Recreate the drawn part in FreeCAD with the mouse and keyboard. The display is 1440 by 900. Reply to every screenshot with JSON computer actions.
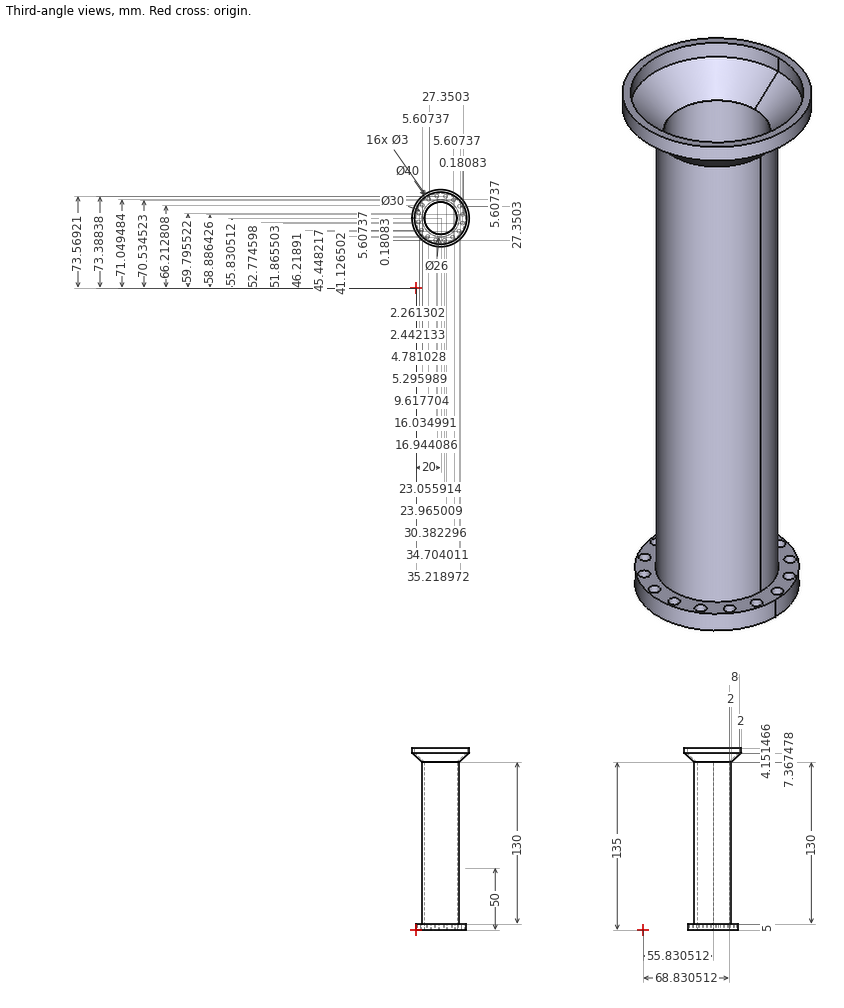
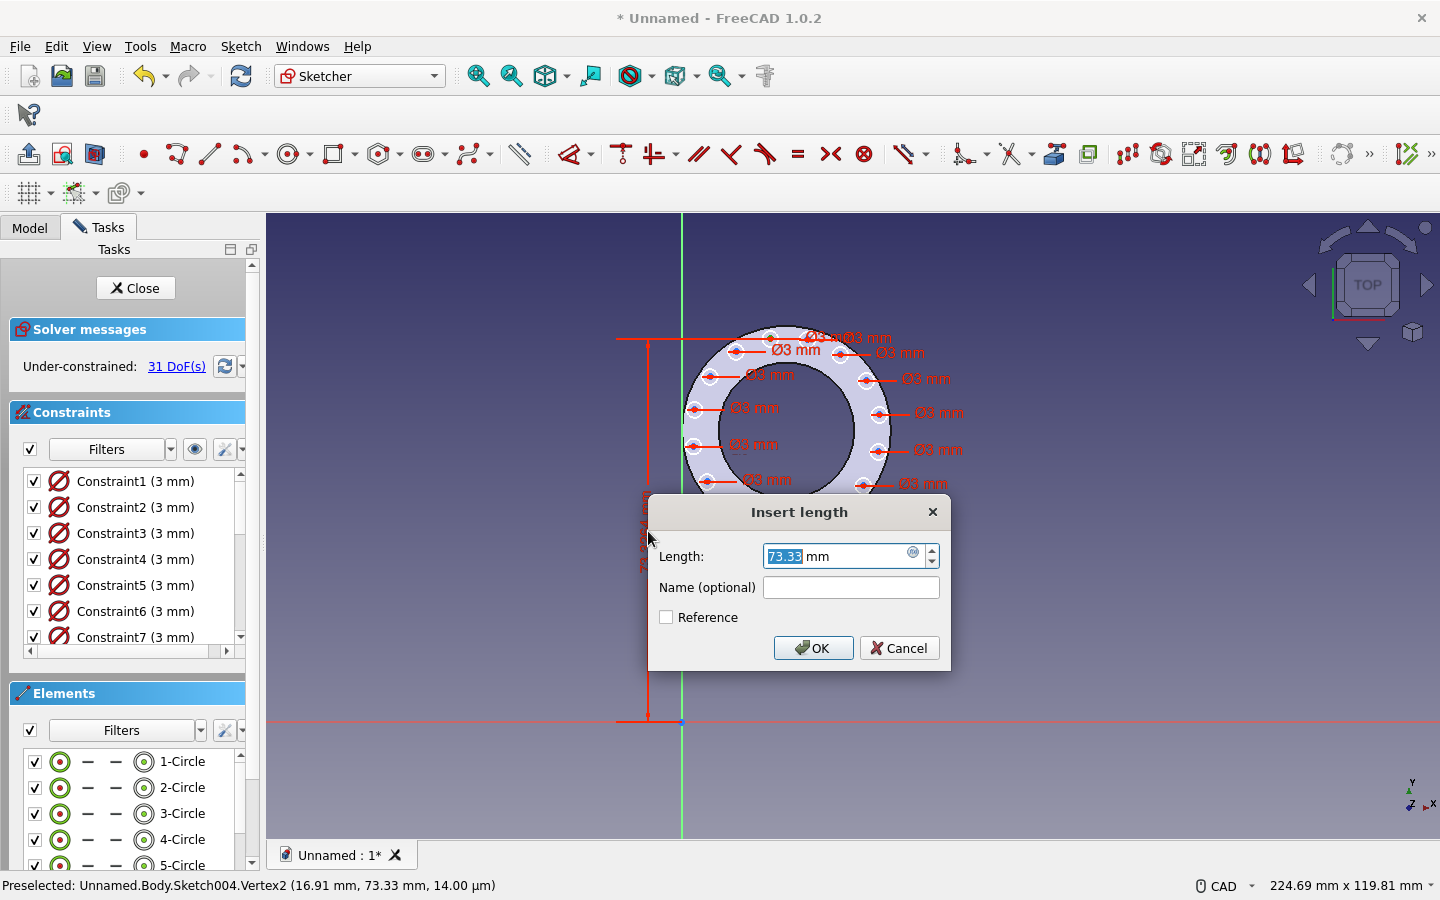
{"action": "type", "text": "73.56921"}
{"action": "key", "text": "Return"}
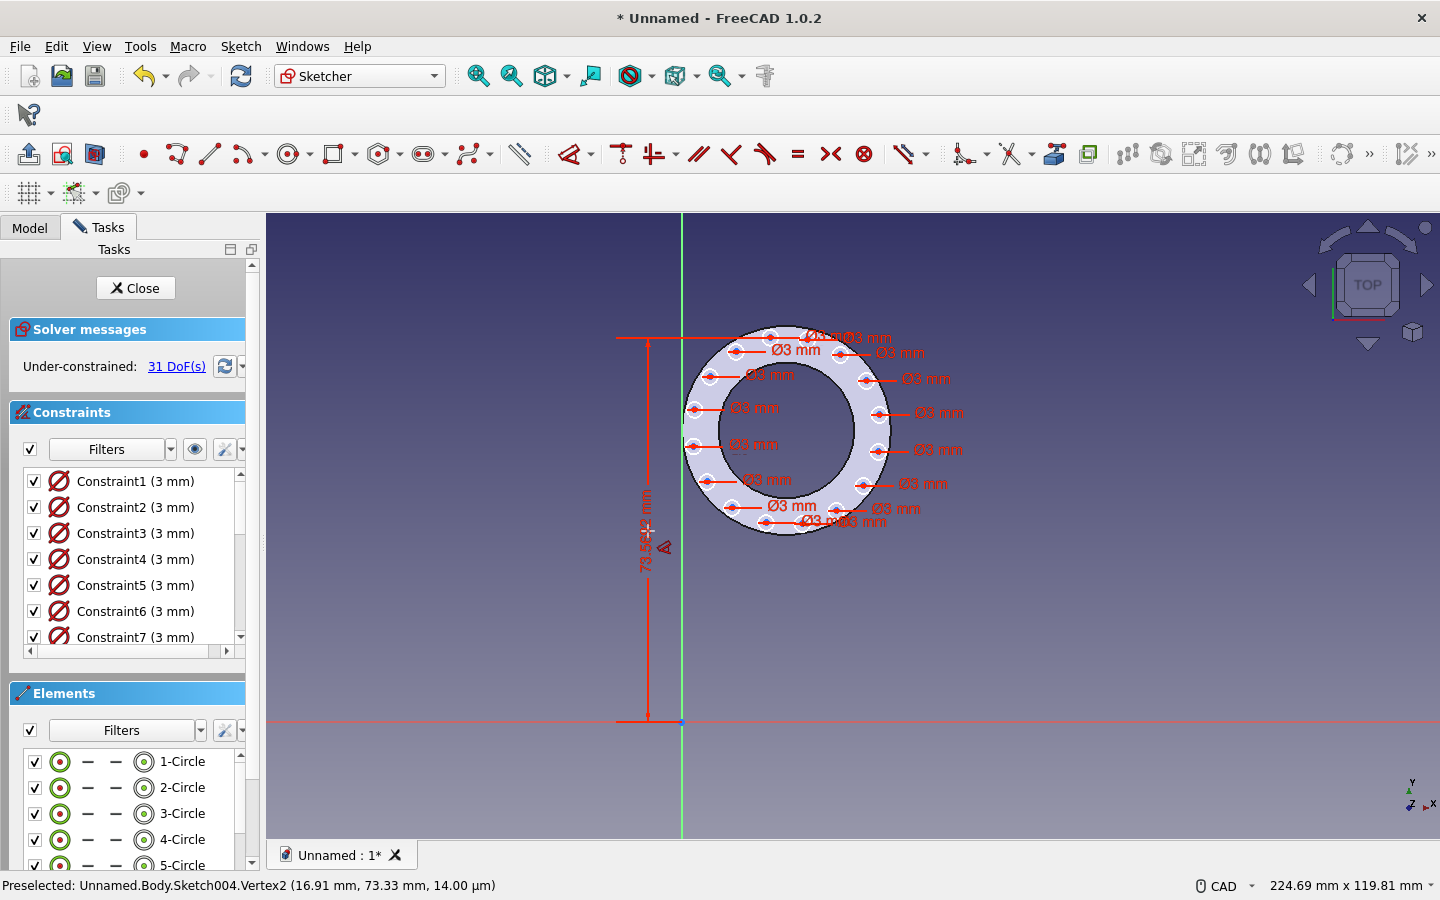
{"action": "left_click", "coordinate": [807, 340]}
{"action": "left_click", "coordinate": [648, 443]}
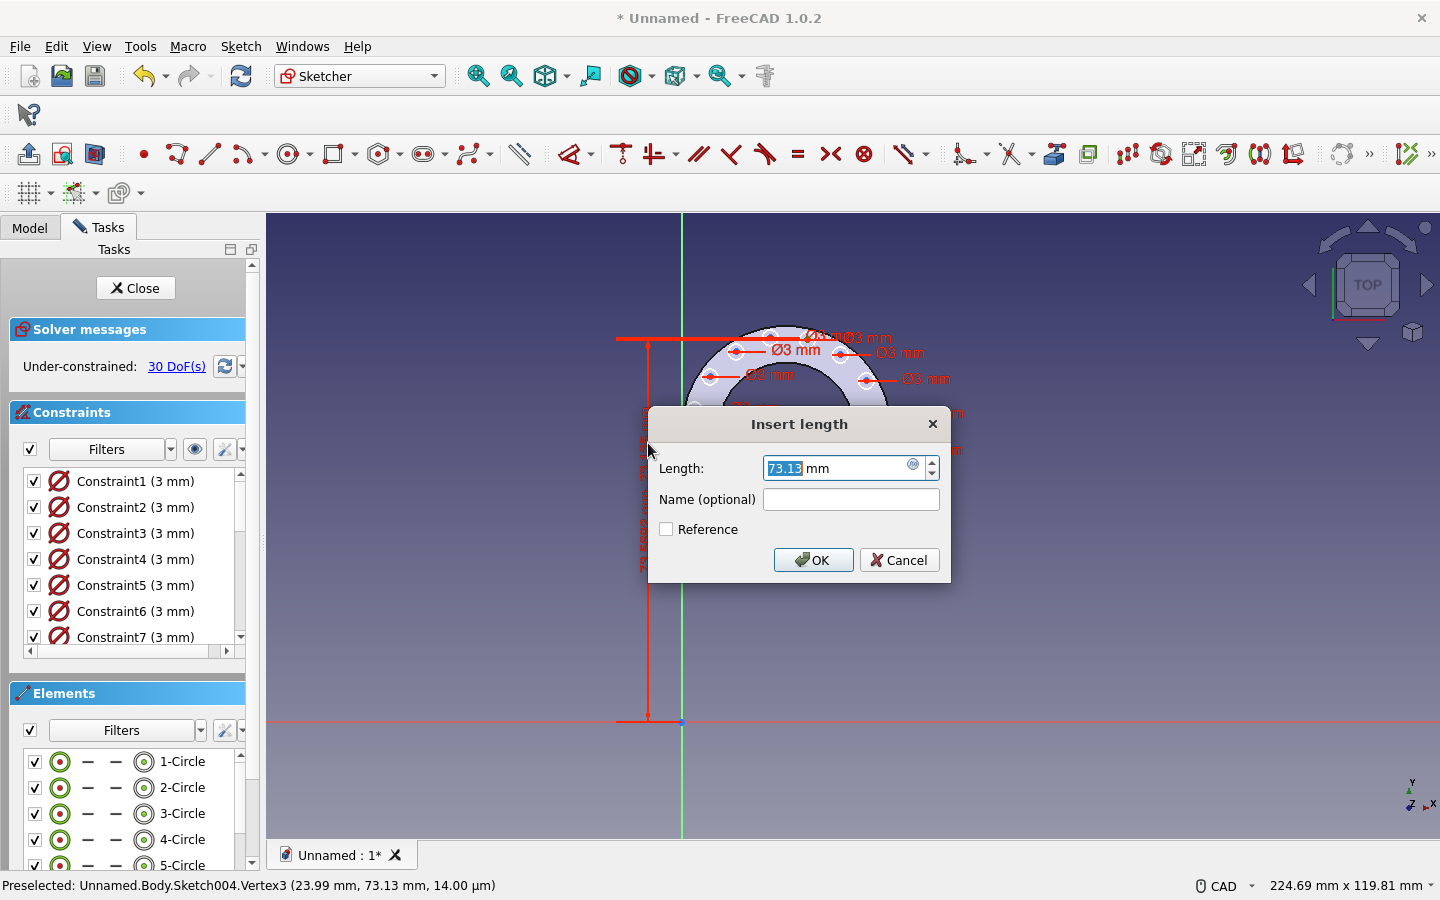
{"action": "type", "text": "73.38838"}
{"action": "key", "text": "Return"}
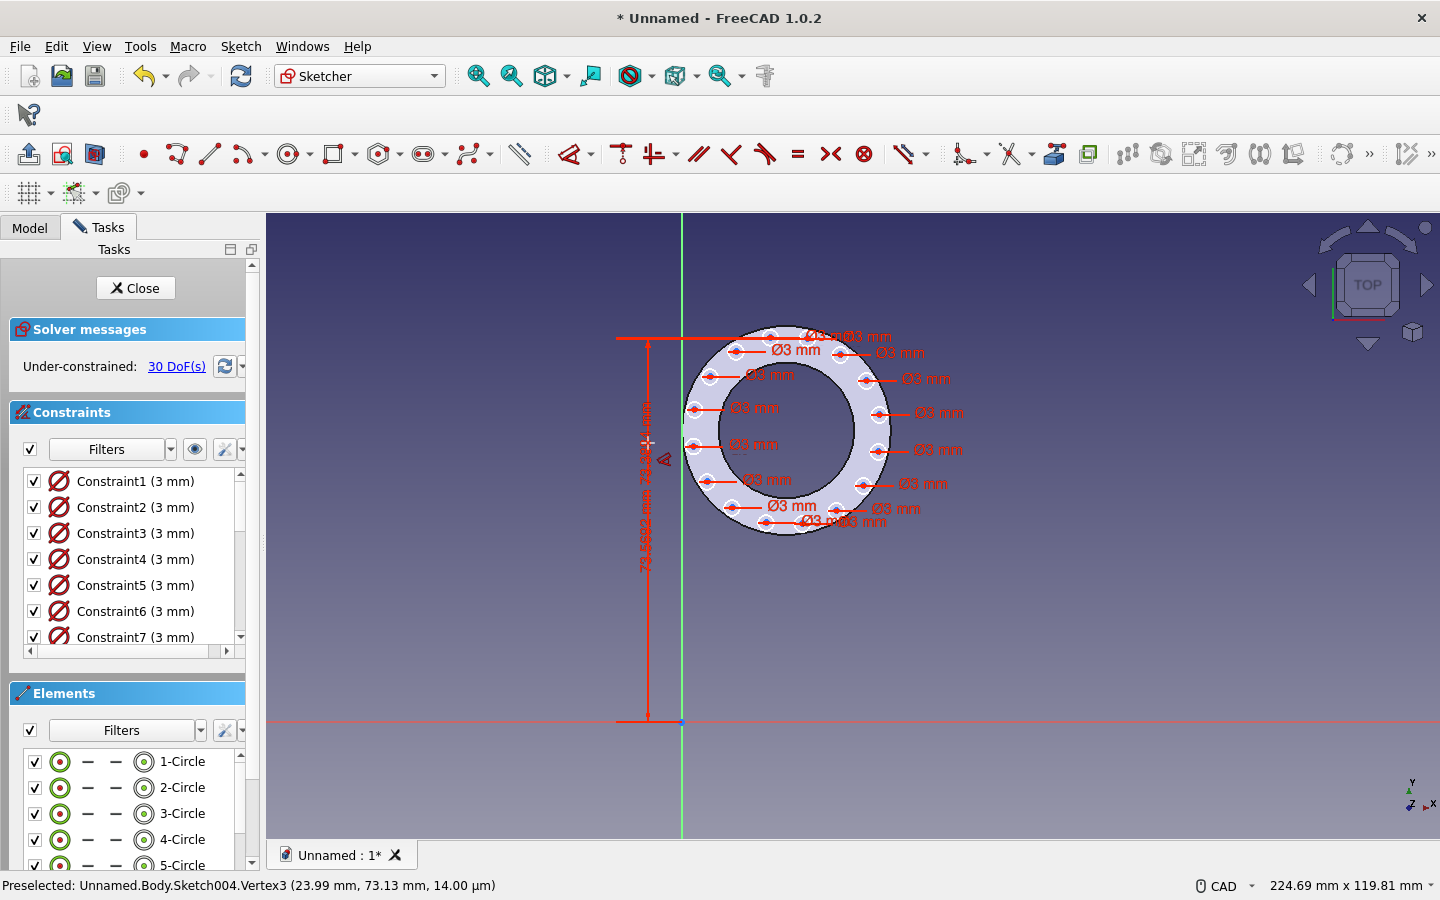
{"action": "left_click", "coordinate": [732, 508]}
{"action": "left_click", "coordinate": [707, 756]}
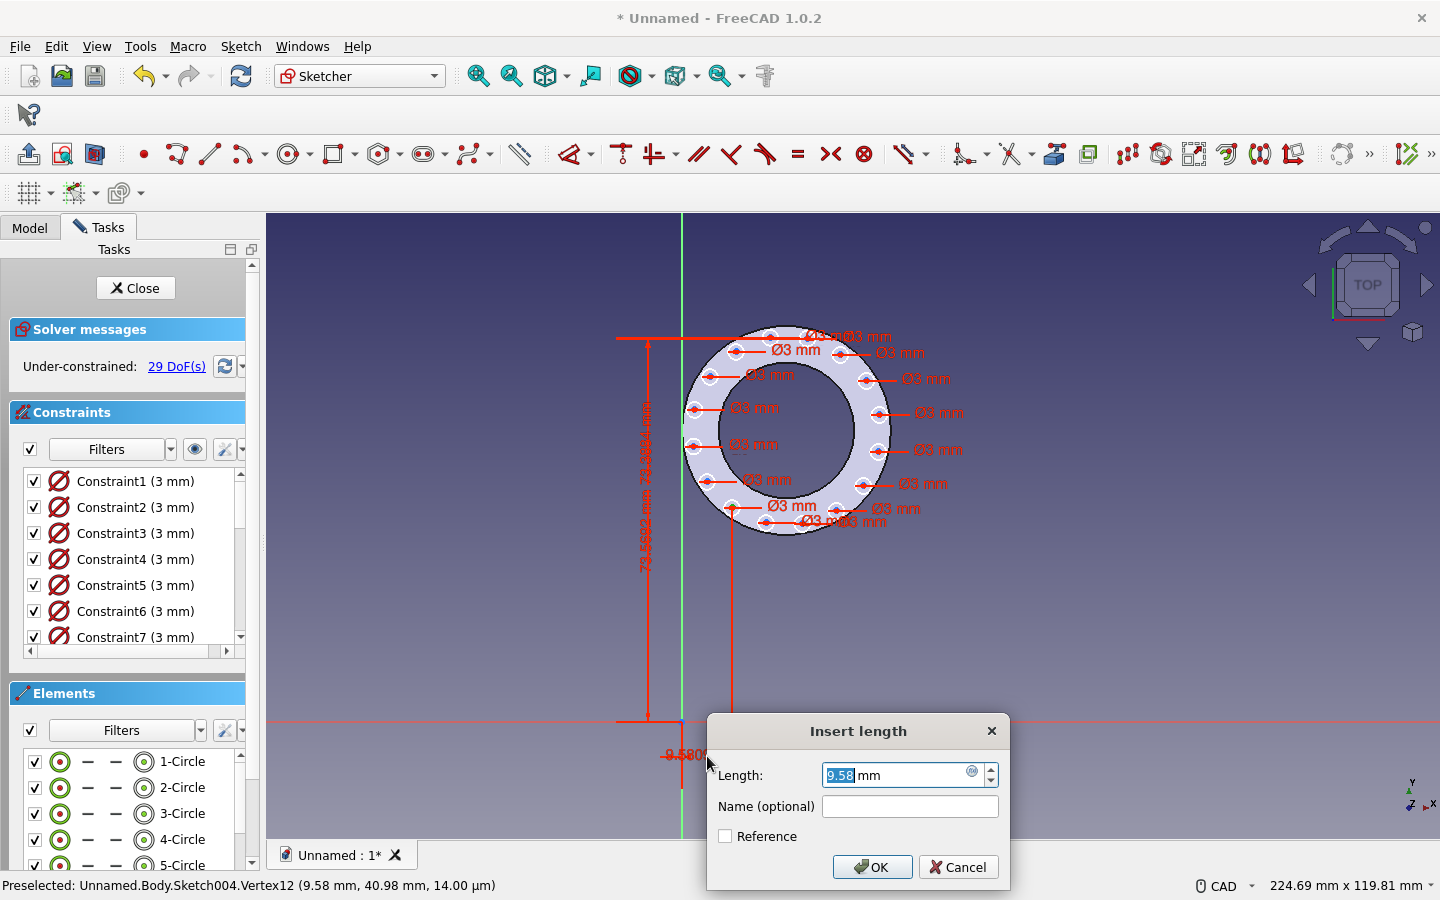
{"action": "type", "text": "9.617704"}
{"action": "key", "text": "Return"}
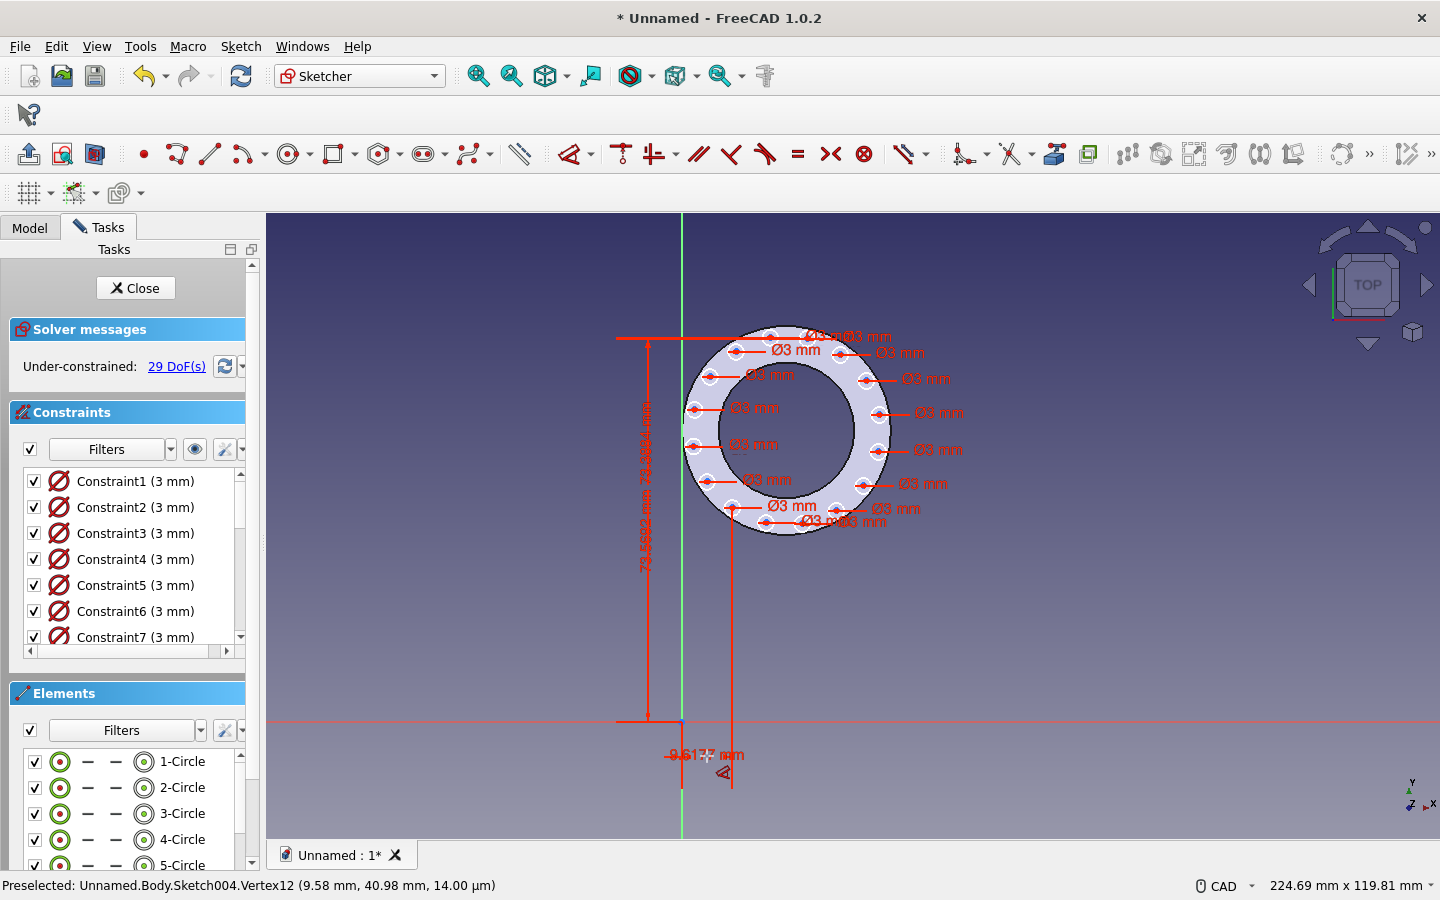
{"action": "scroll", "coordinate": [707, 482], "scroll_direction": "up", "scroll_amount": 3}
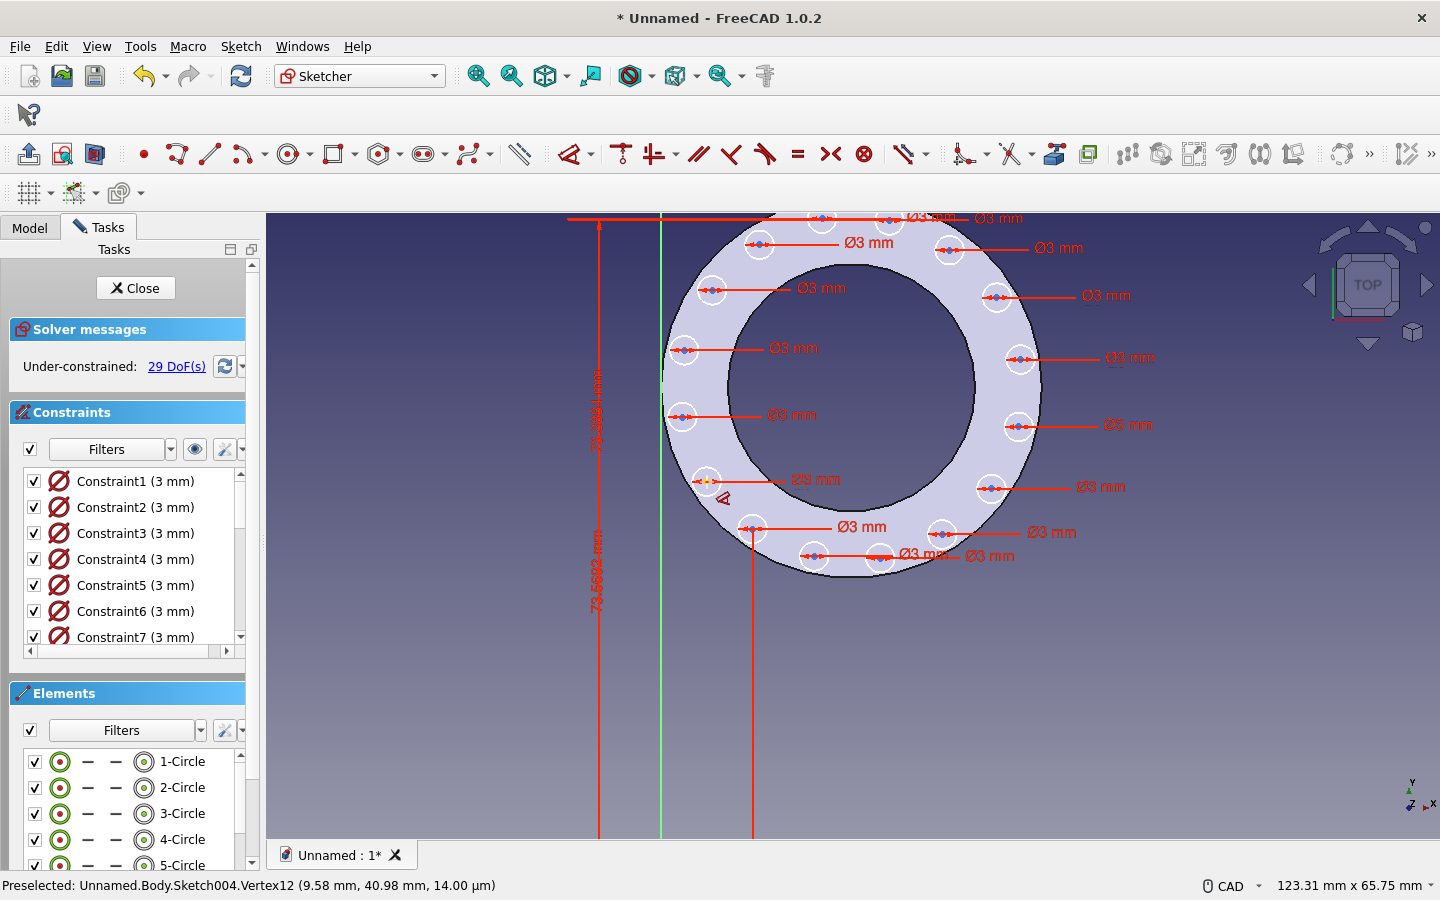
{"action": "left_click", "coordinate": [707, 482]}
{"action": "left_click", "coordinate": [684, 448]}